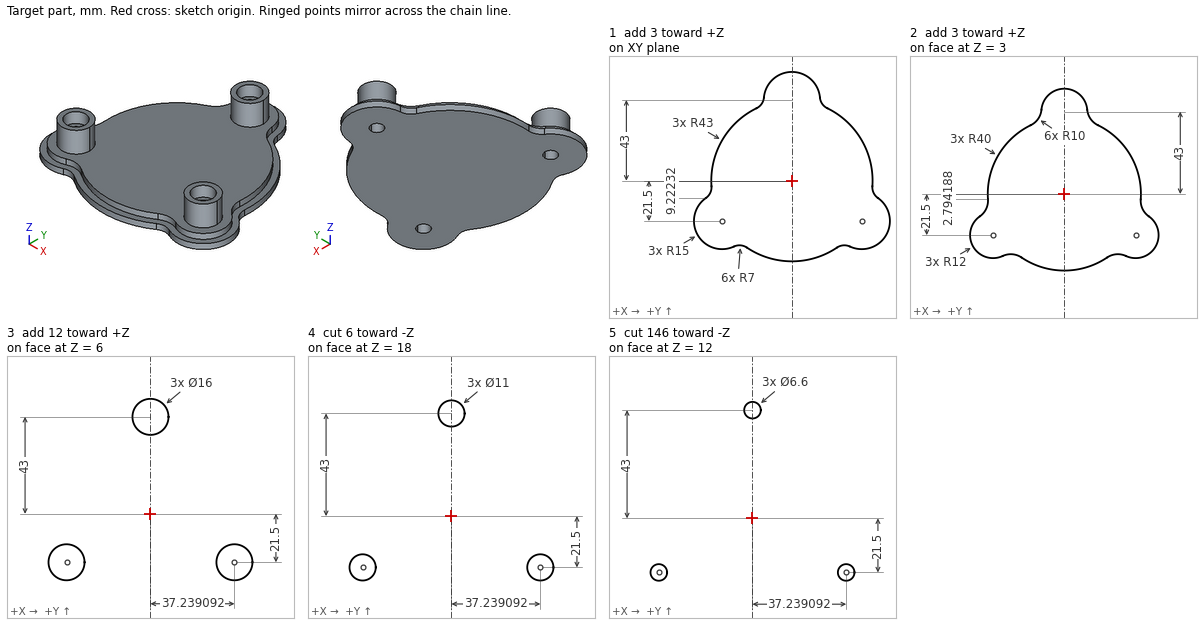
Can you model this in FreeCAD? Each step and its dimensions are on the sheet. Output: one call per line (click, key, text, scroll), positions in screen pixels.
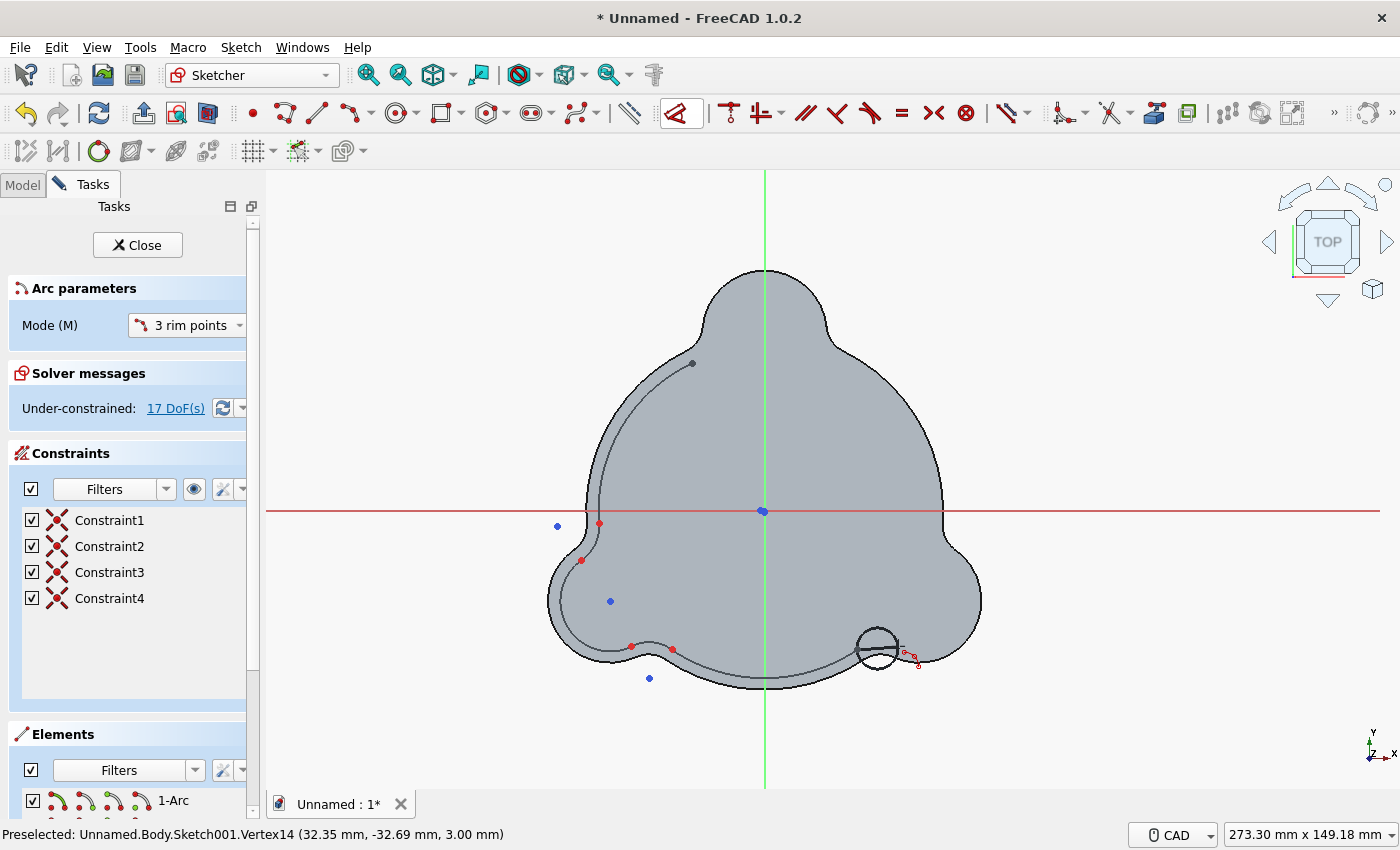
scroll(877, 642, up, 6)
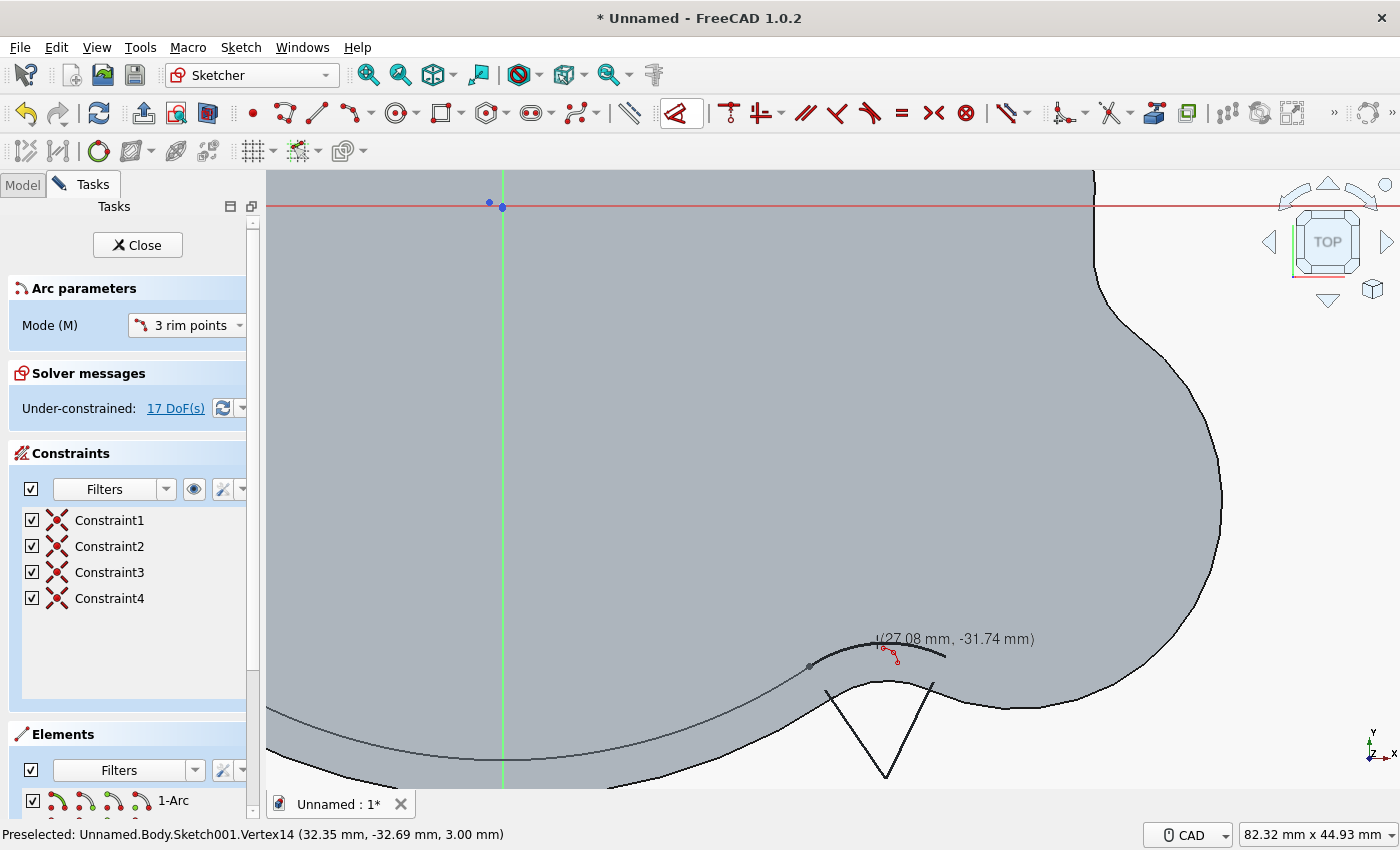
click(877, 640)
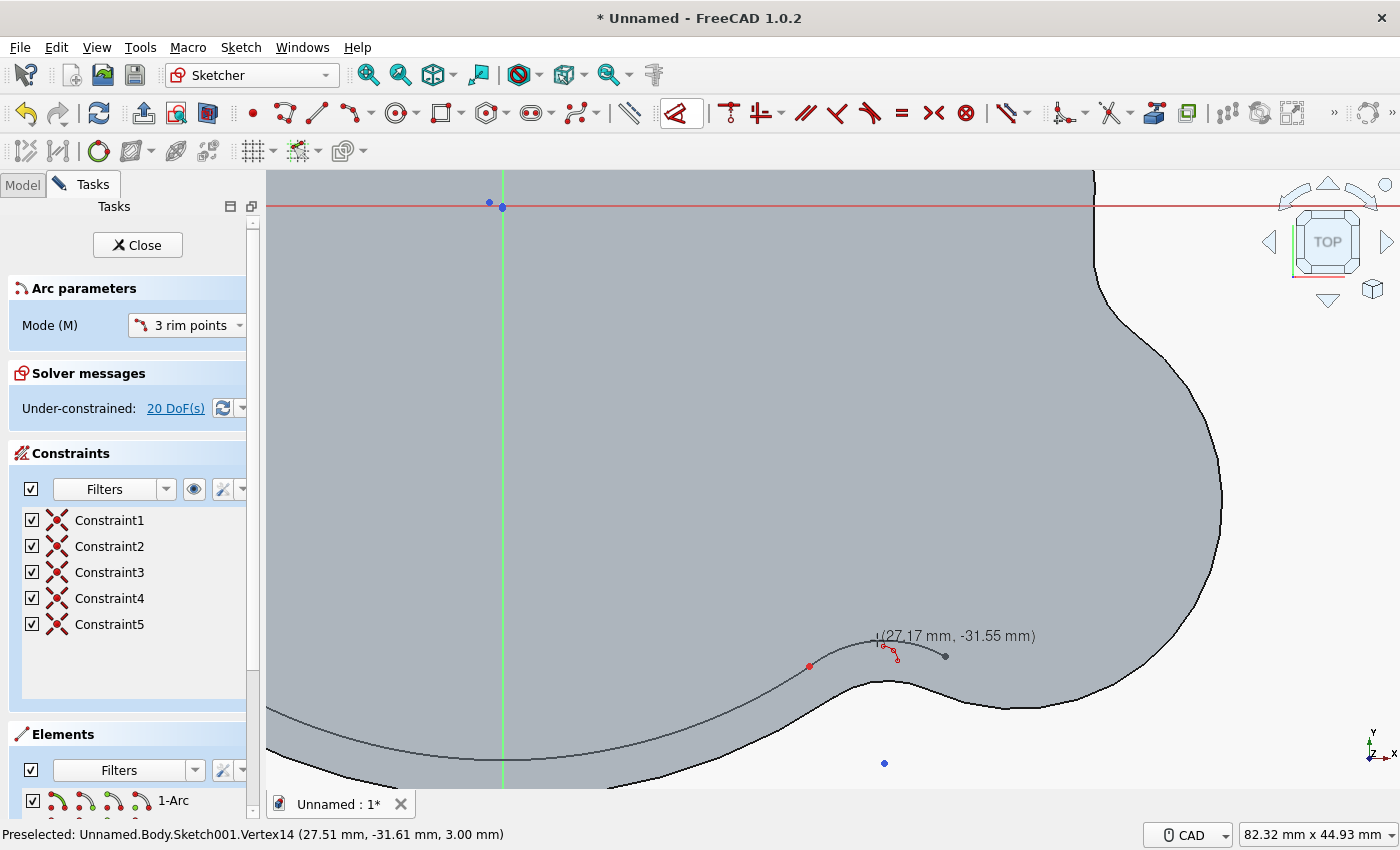
click(945, 657)
click(1111, 367)
click(1159, 585)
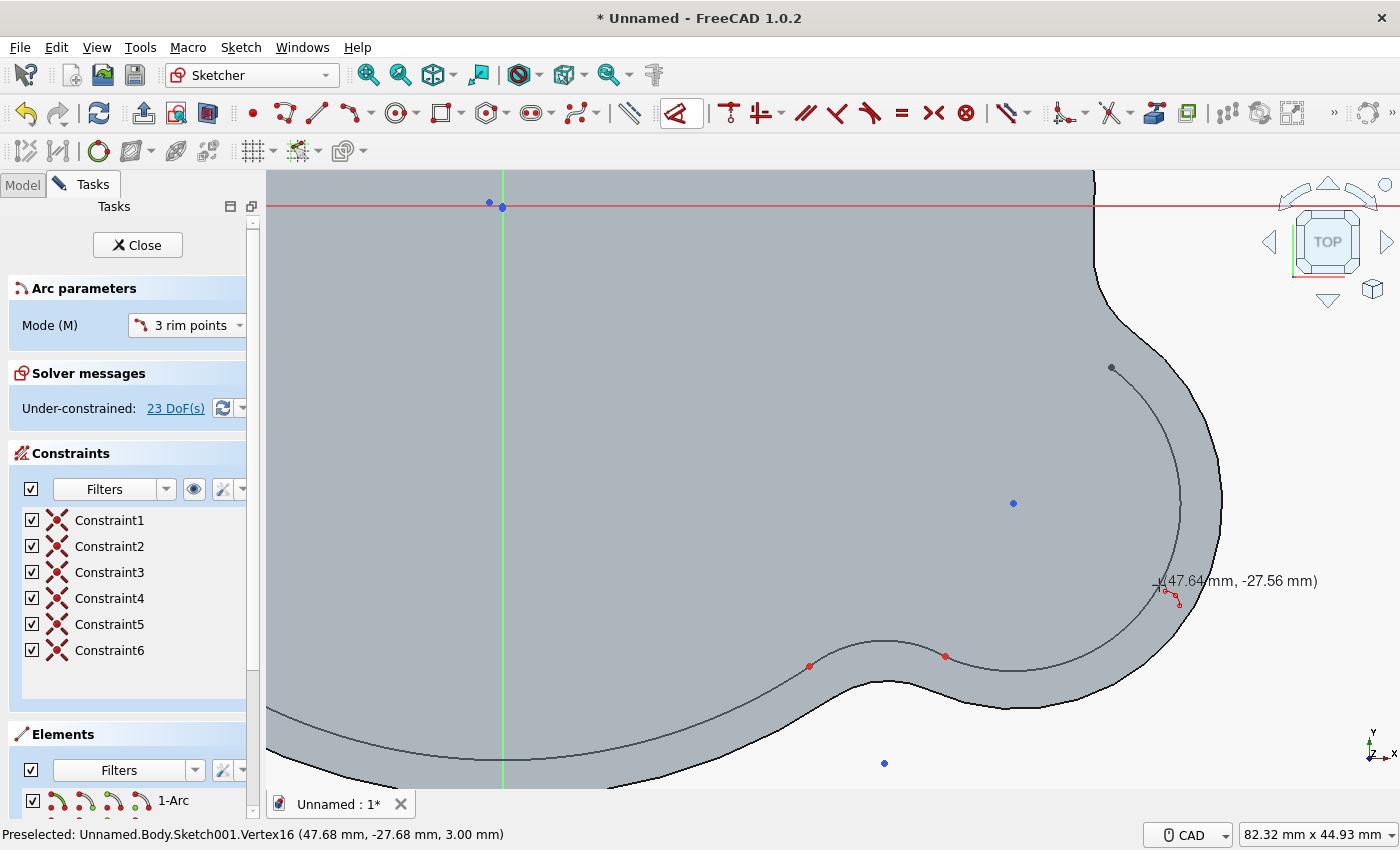
click(1111, 368)
click(1052, 245)
click(1065, 314)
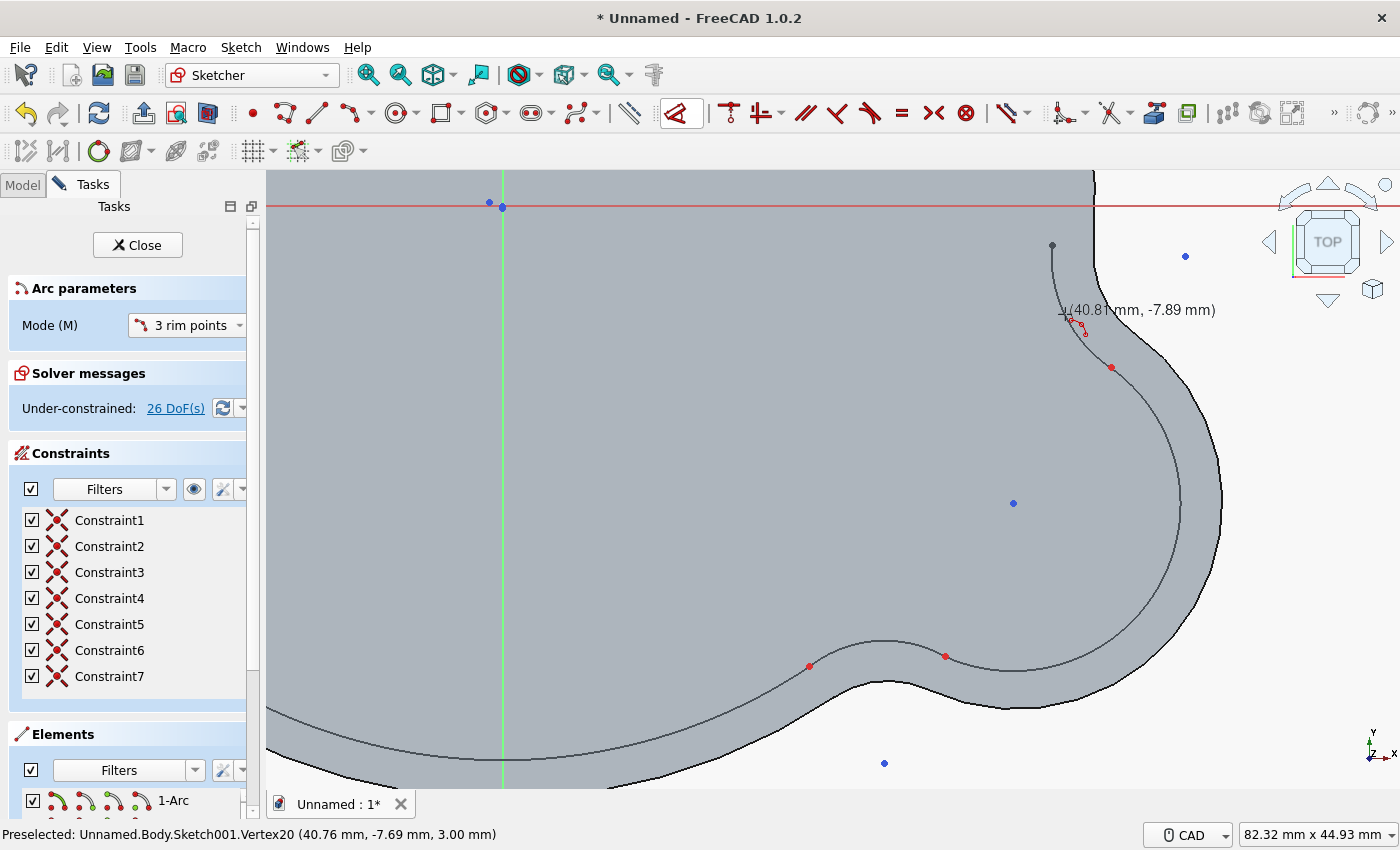
click(1052, 246)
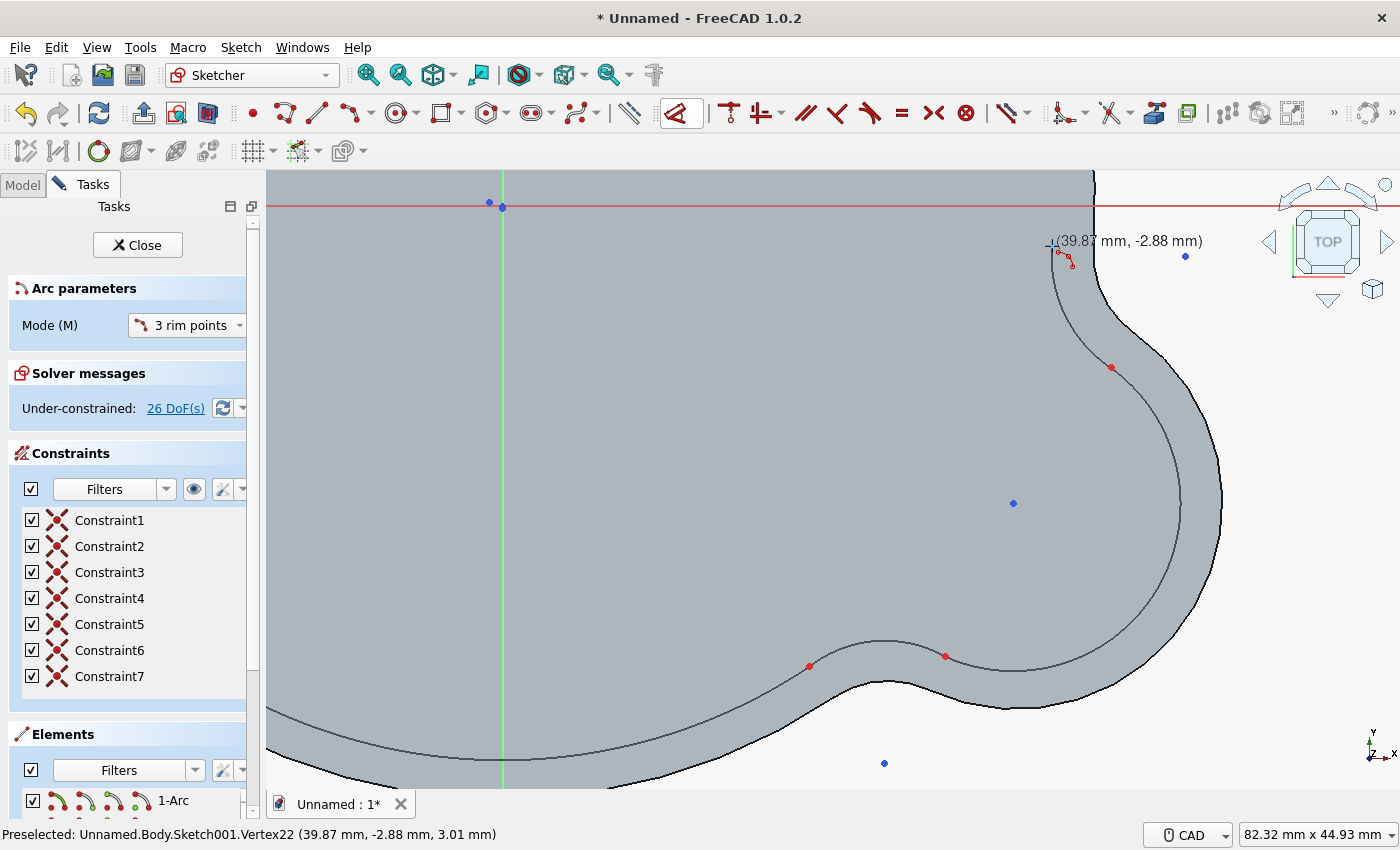
scroll(877, 642, down, 6)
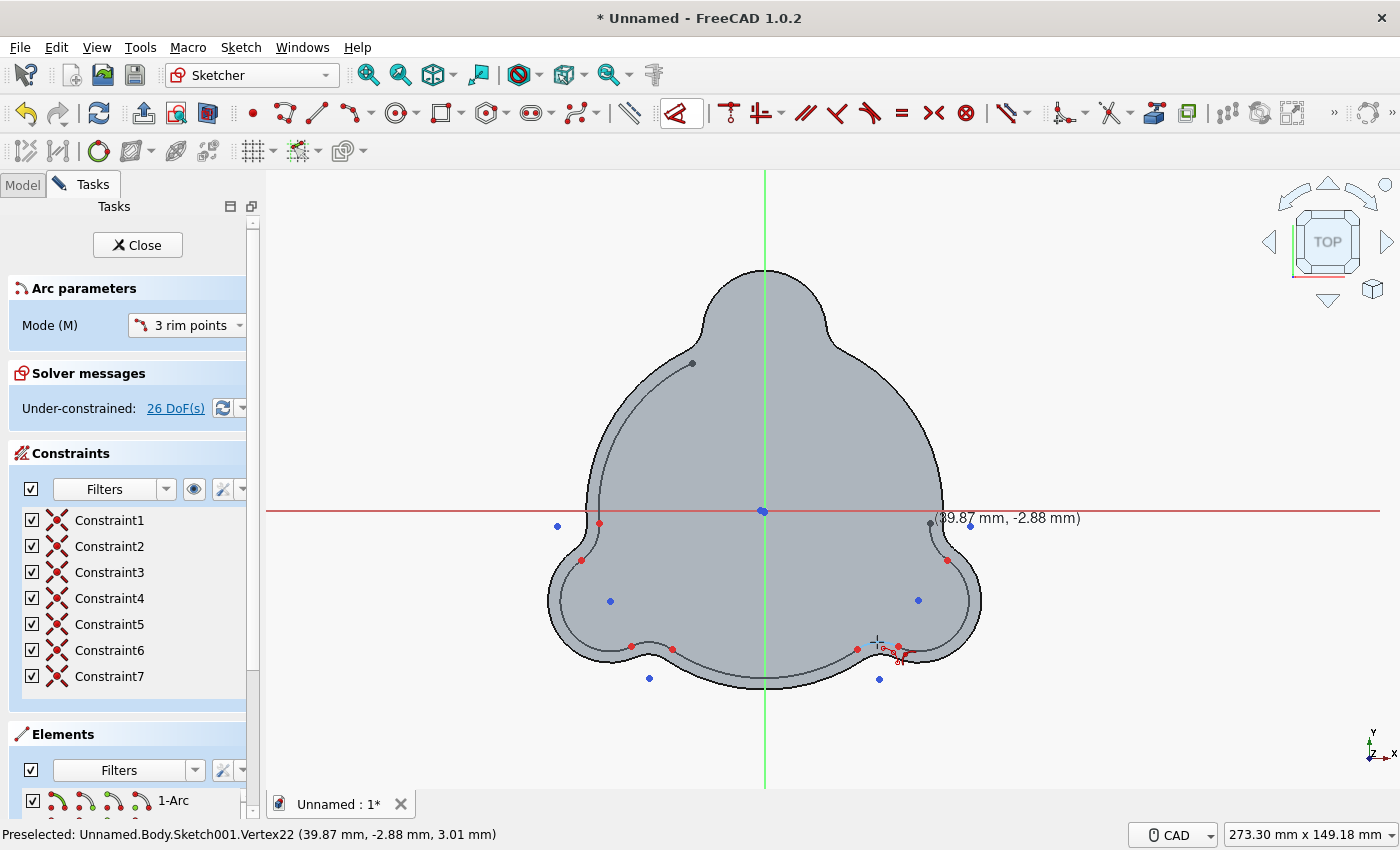
click(837, 362)
click(908, 428)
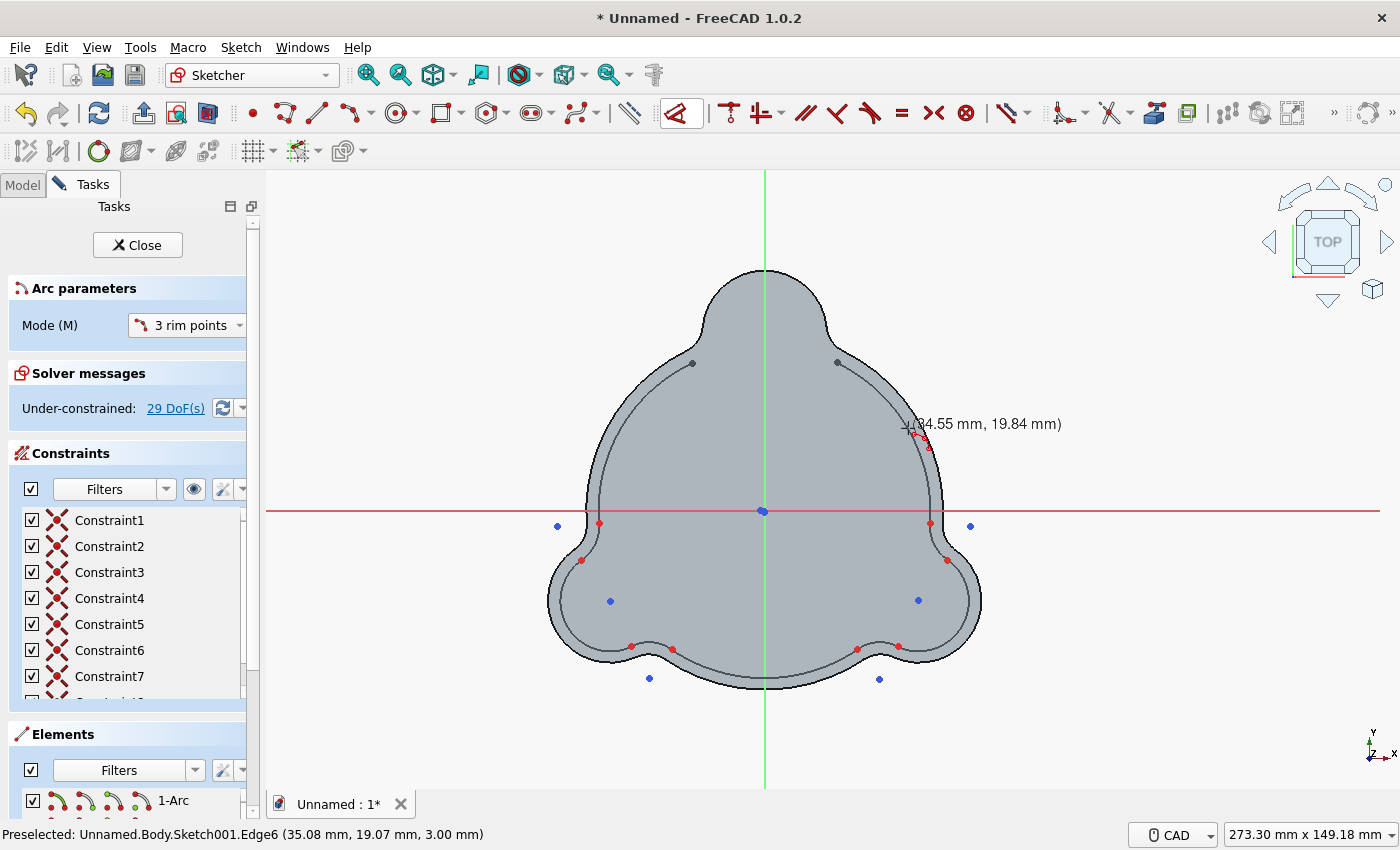
click(837, 363)
click(814, 328)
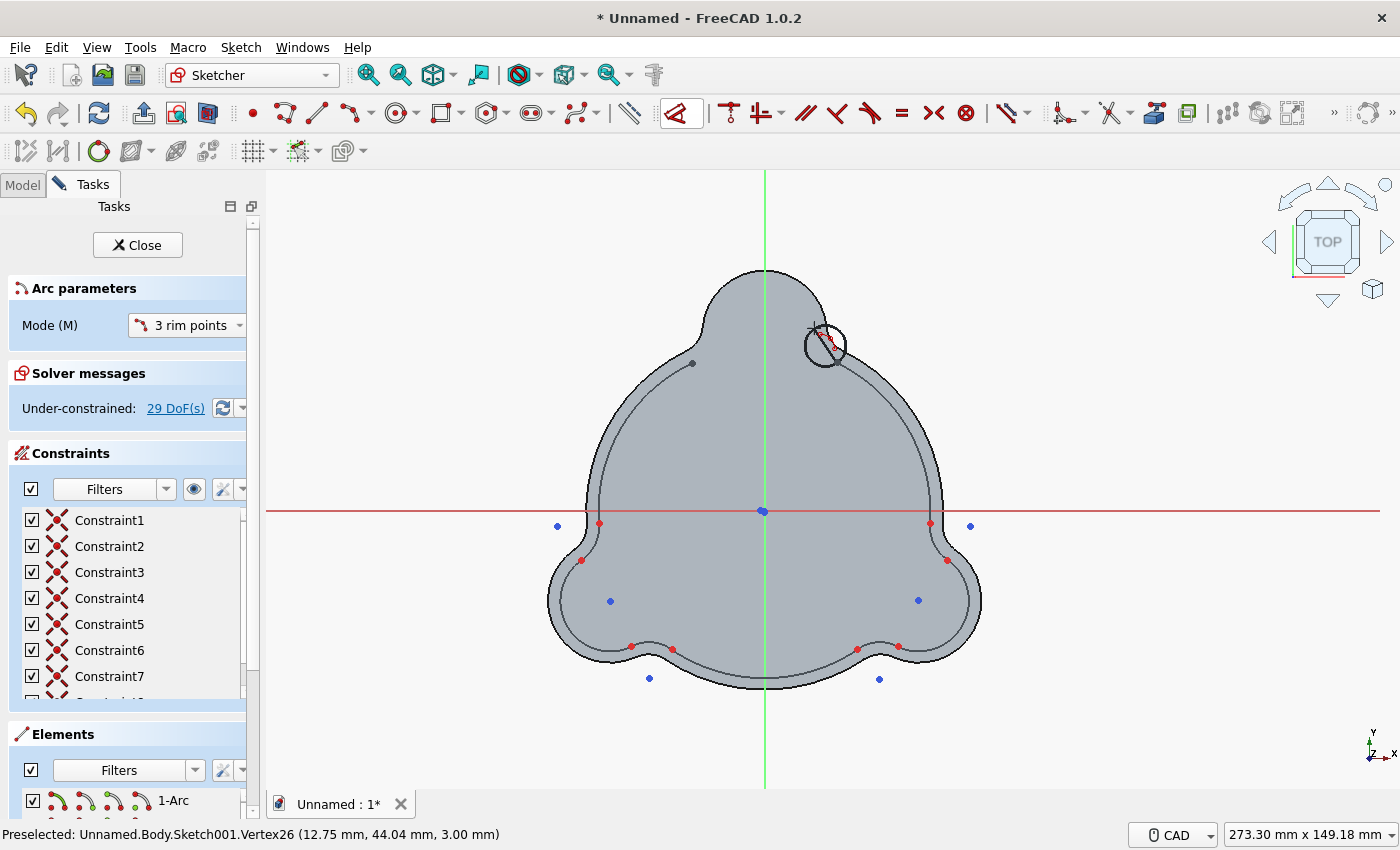
scroll(821, 348, up, 6)